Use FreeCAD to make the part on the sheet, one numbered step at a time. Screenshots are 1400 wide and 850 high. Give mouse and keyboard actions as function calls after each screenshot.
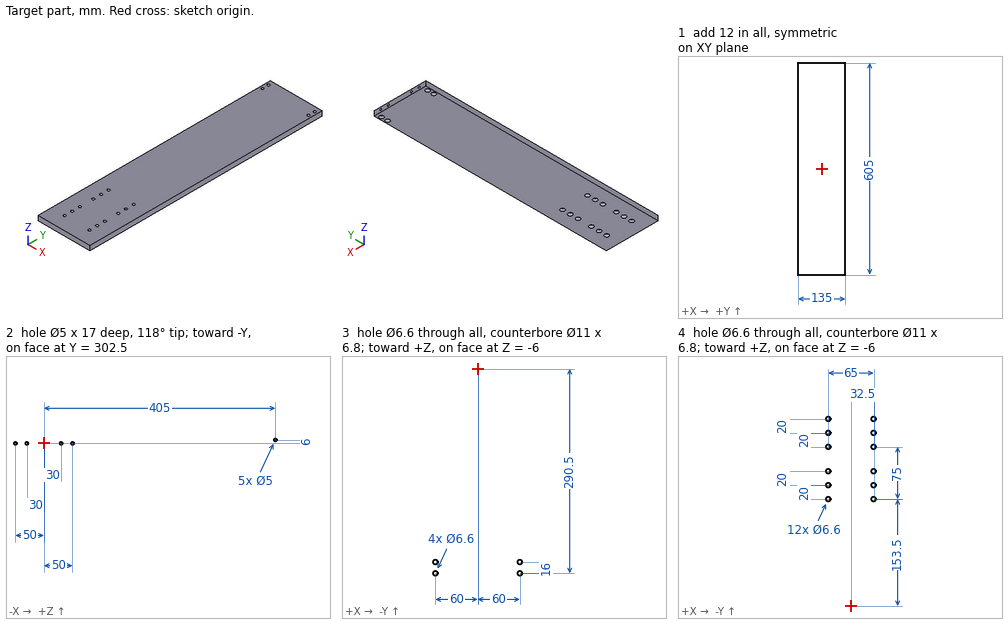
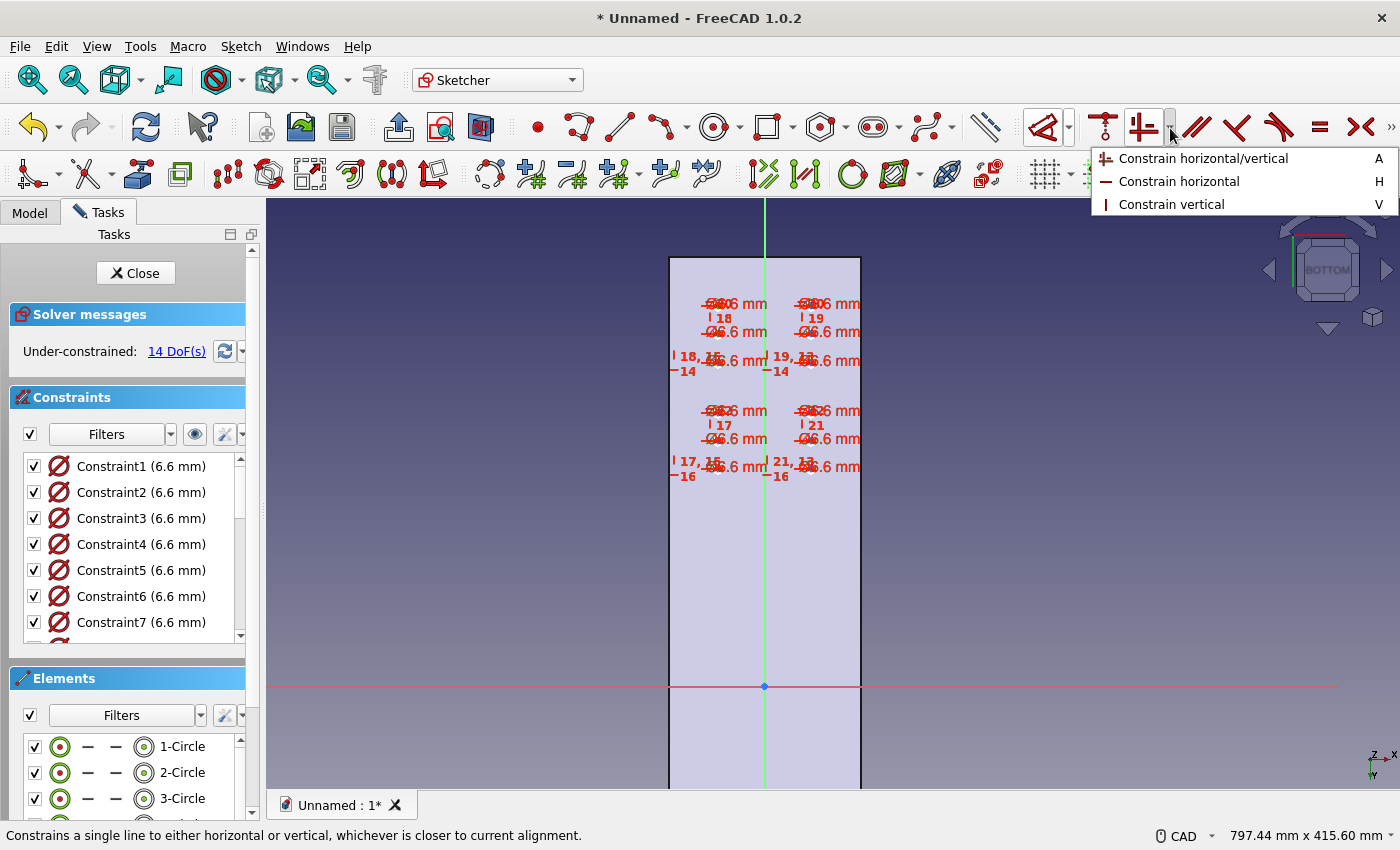
click(1245, 204)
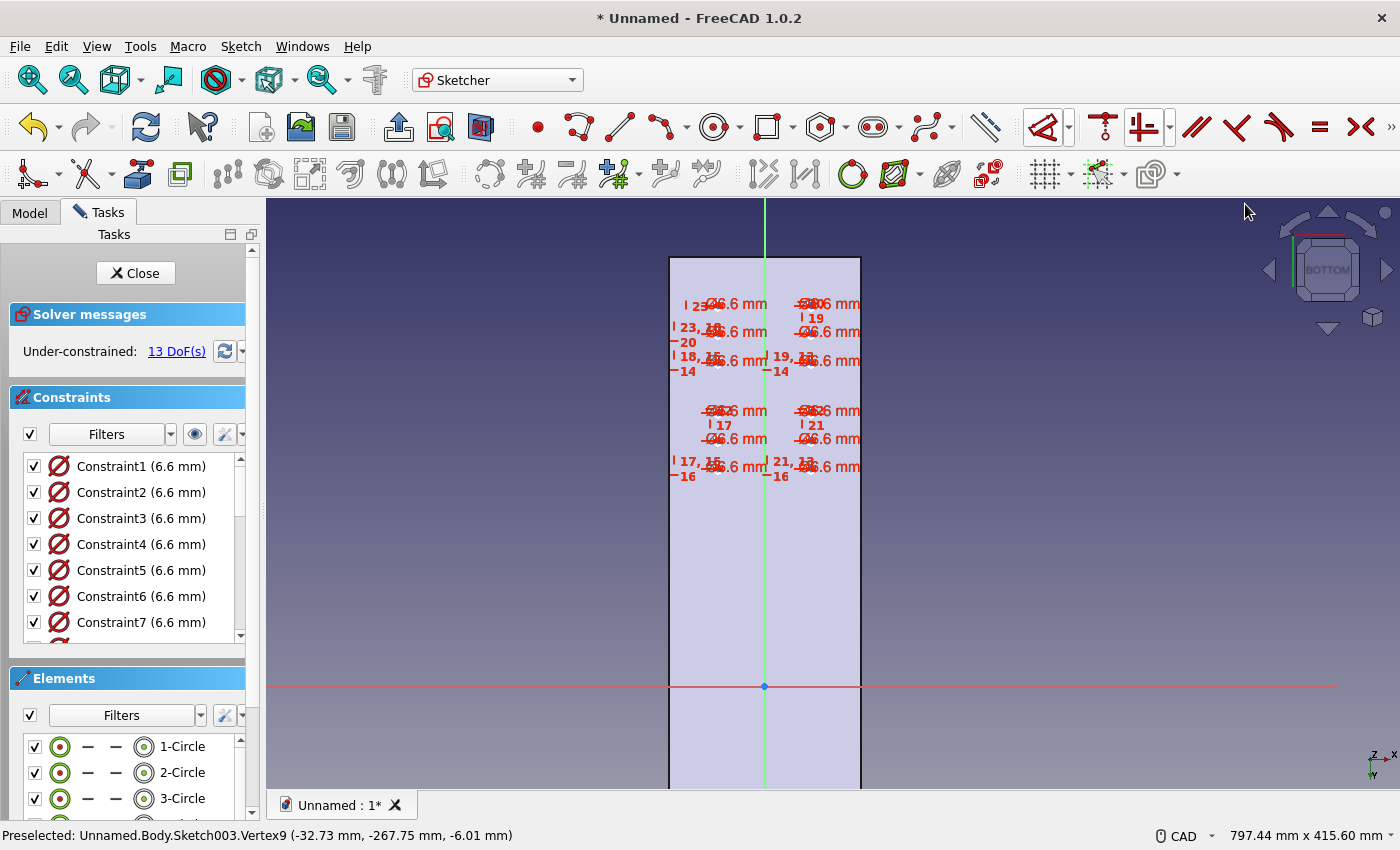
click(718, 441)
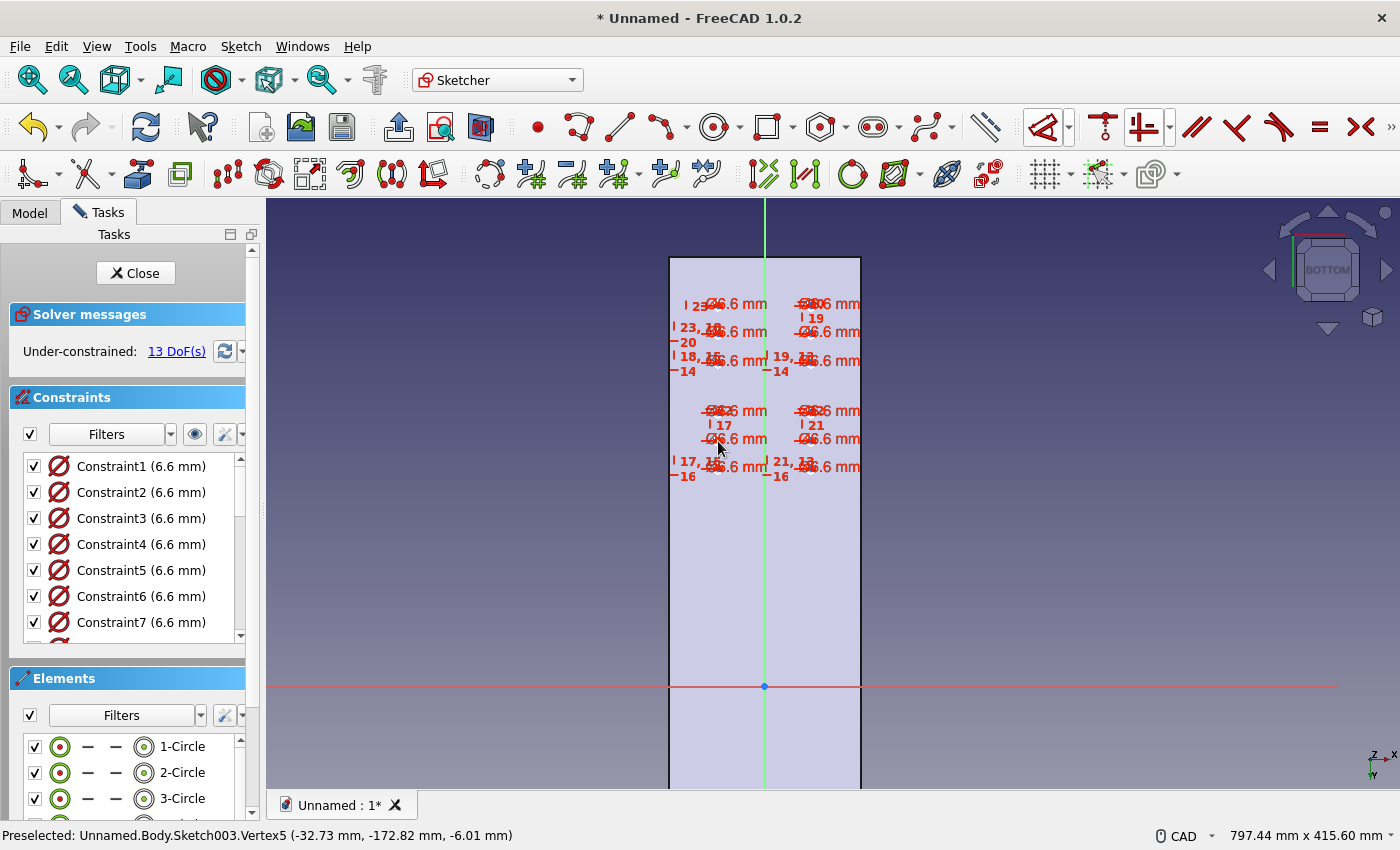
click(718, 413)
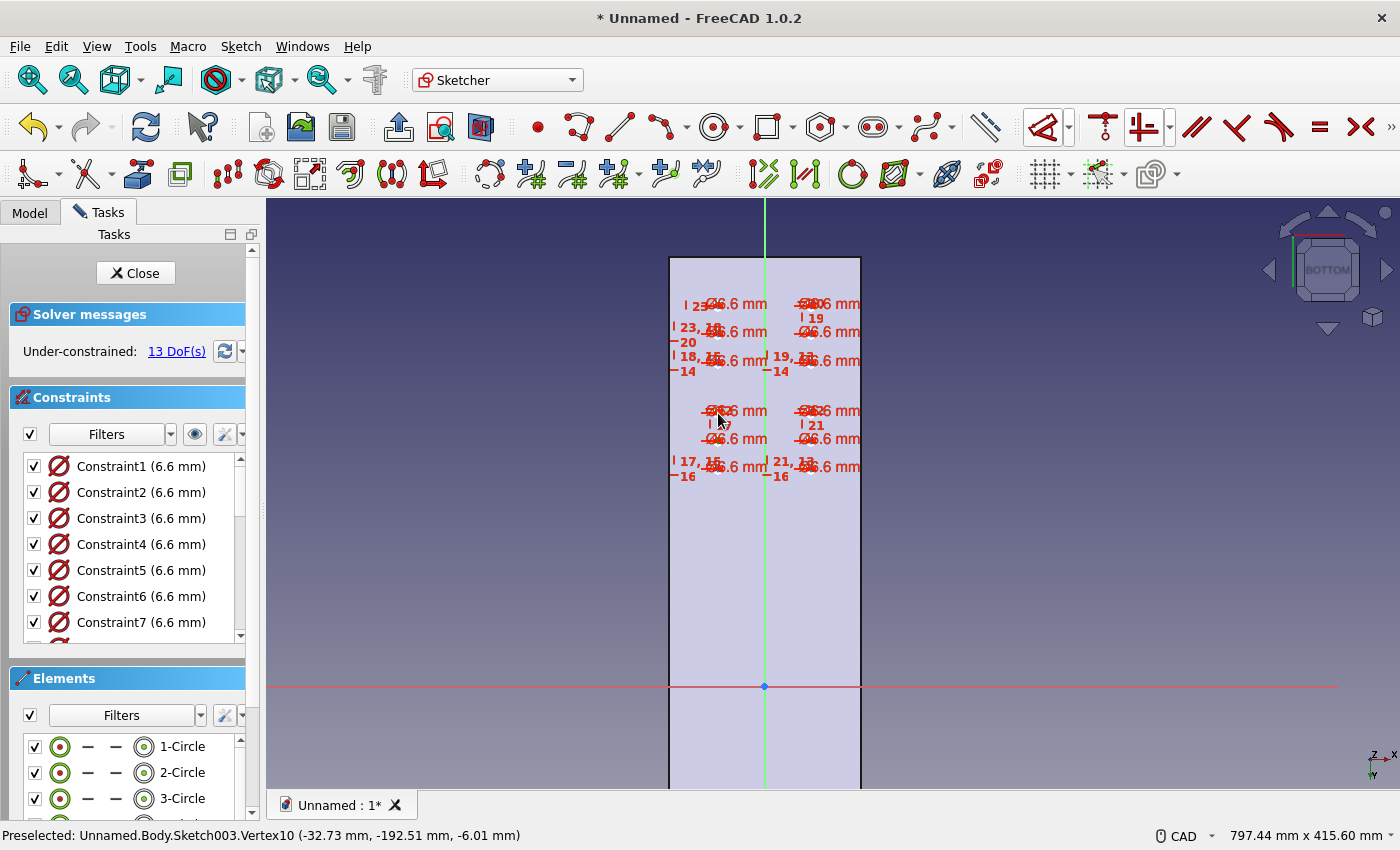
click(1170, 128)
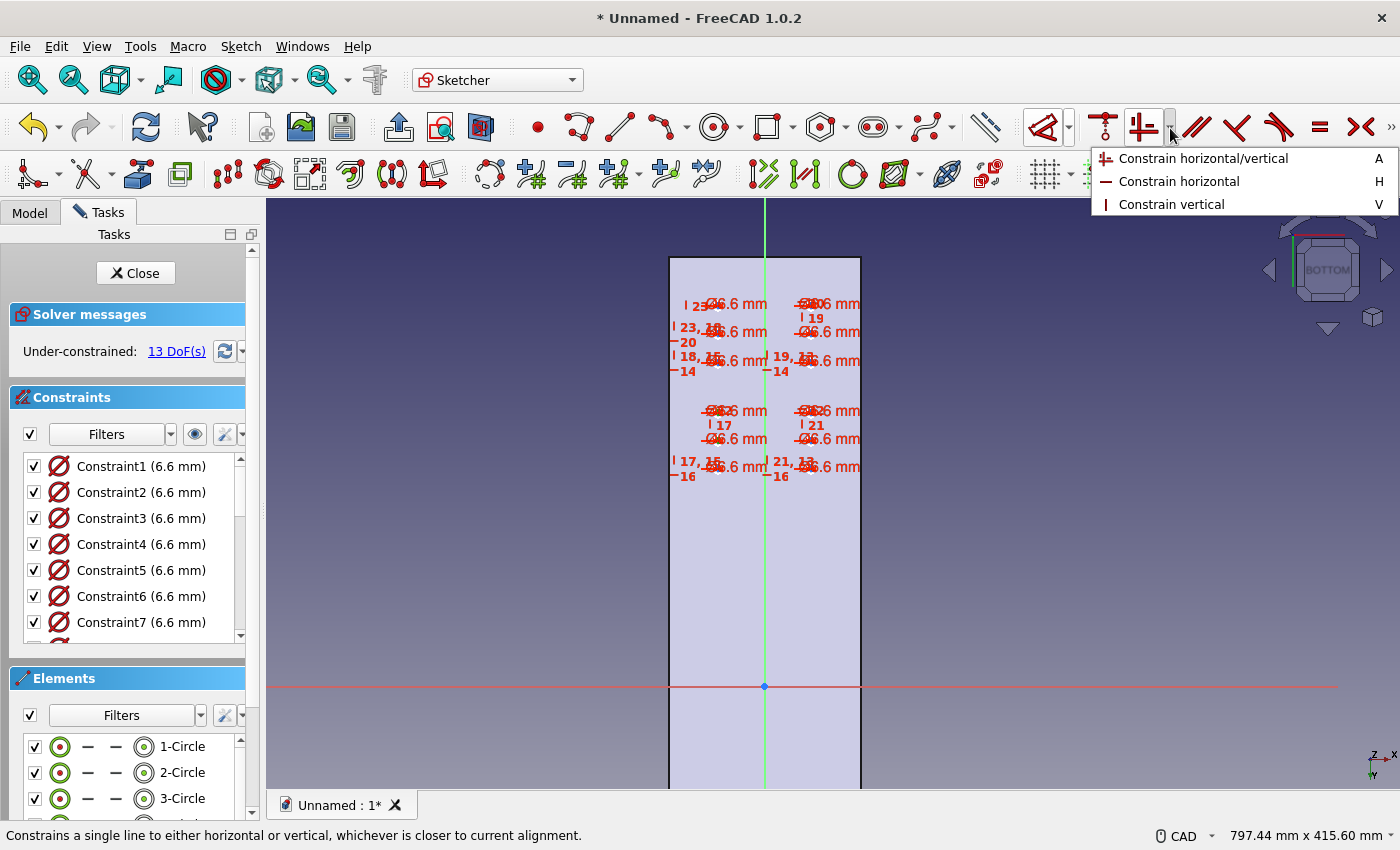
click(1245, 204)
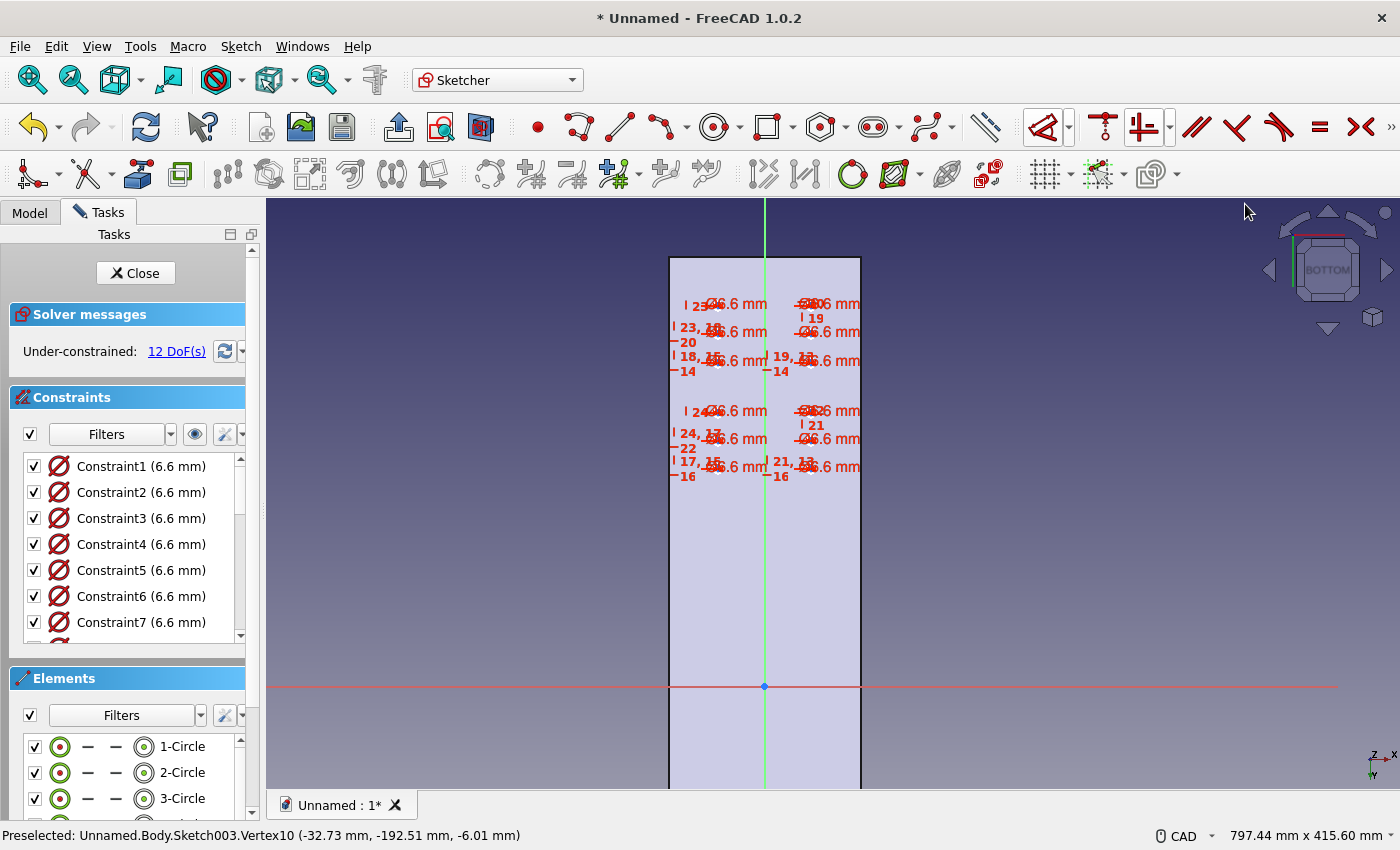
click(811, 441)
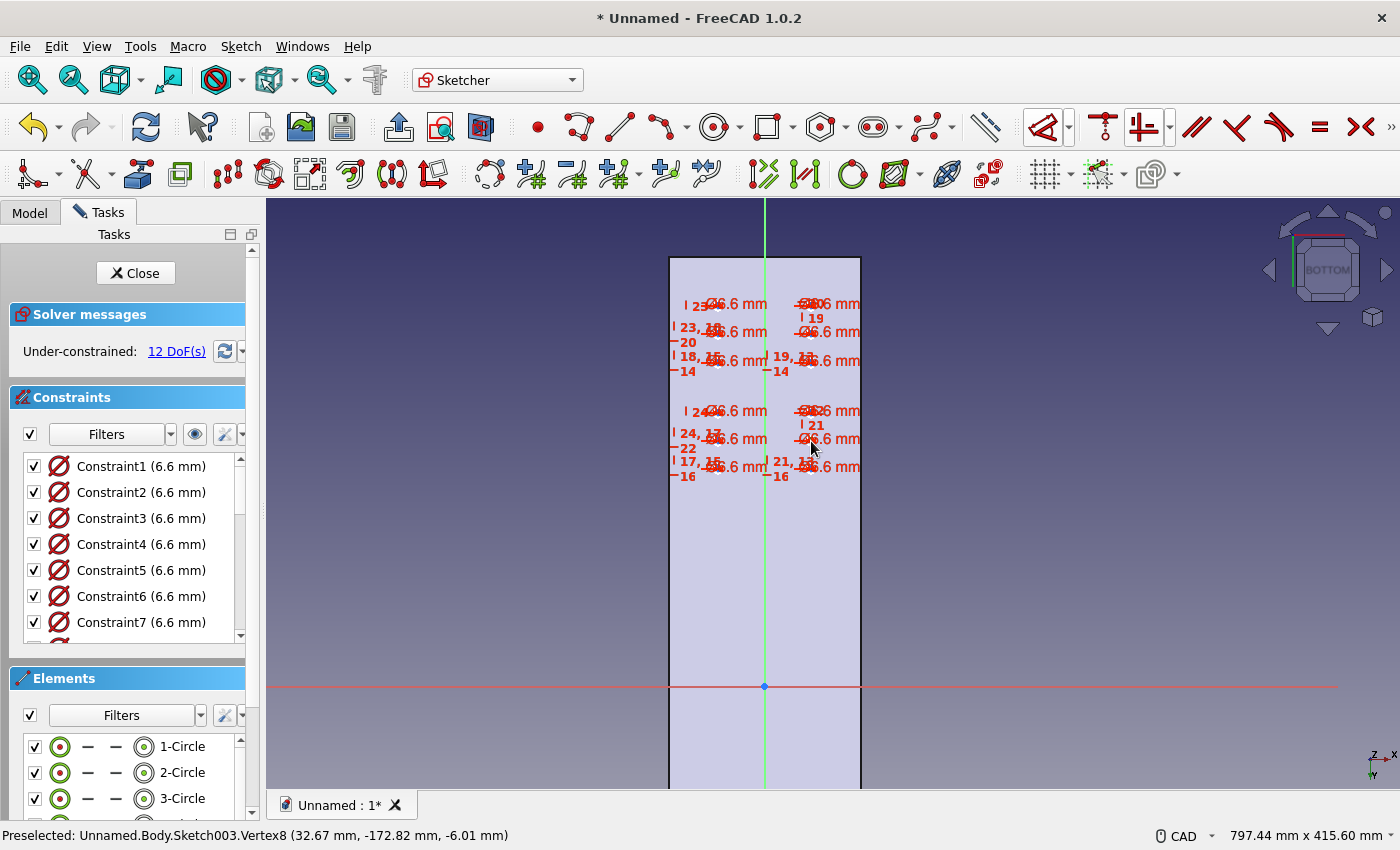
scroll(811, 413, up, 4)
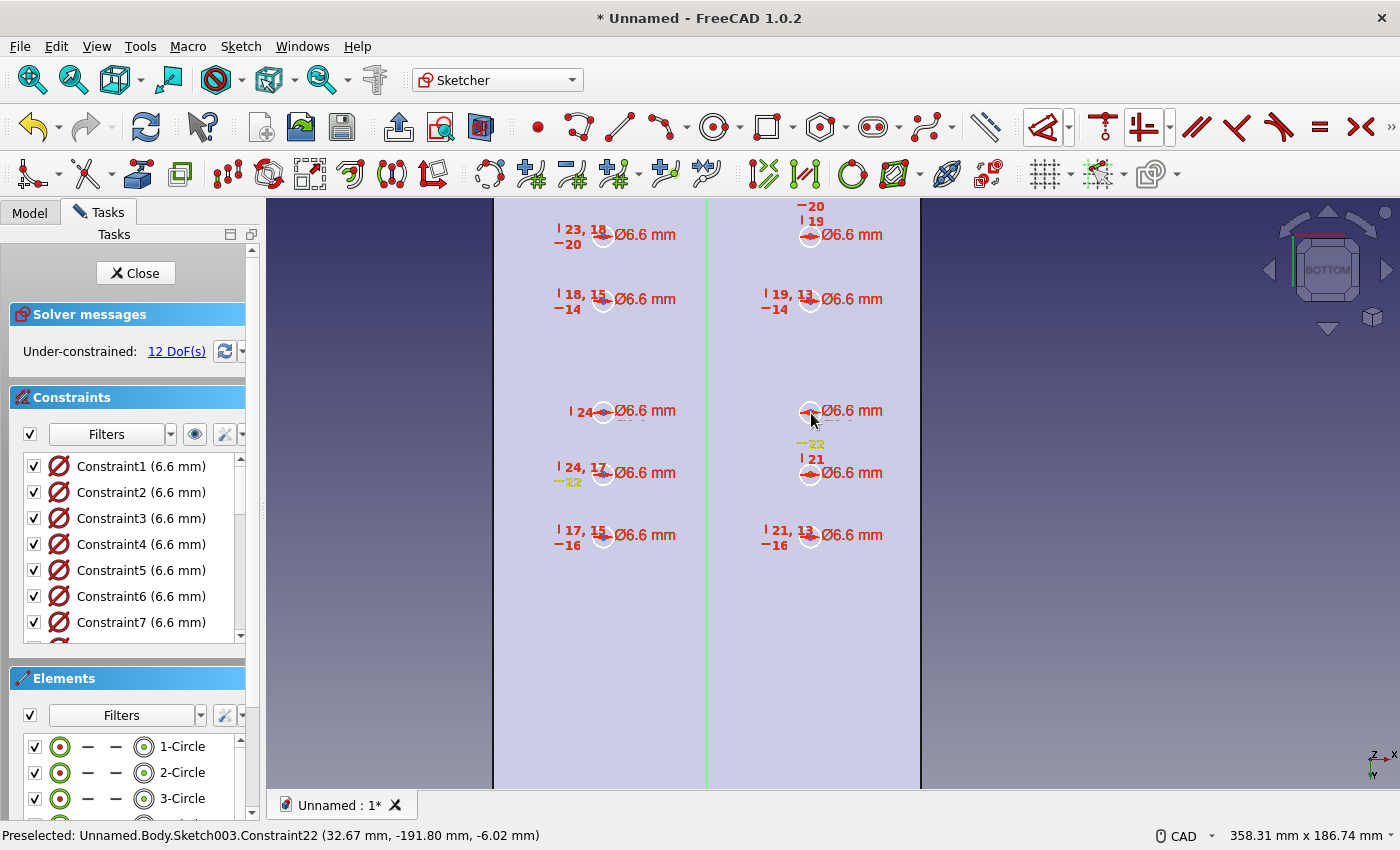
click(810, 413)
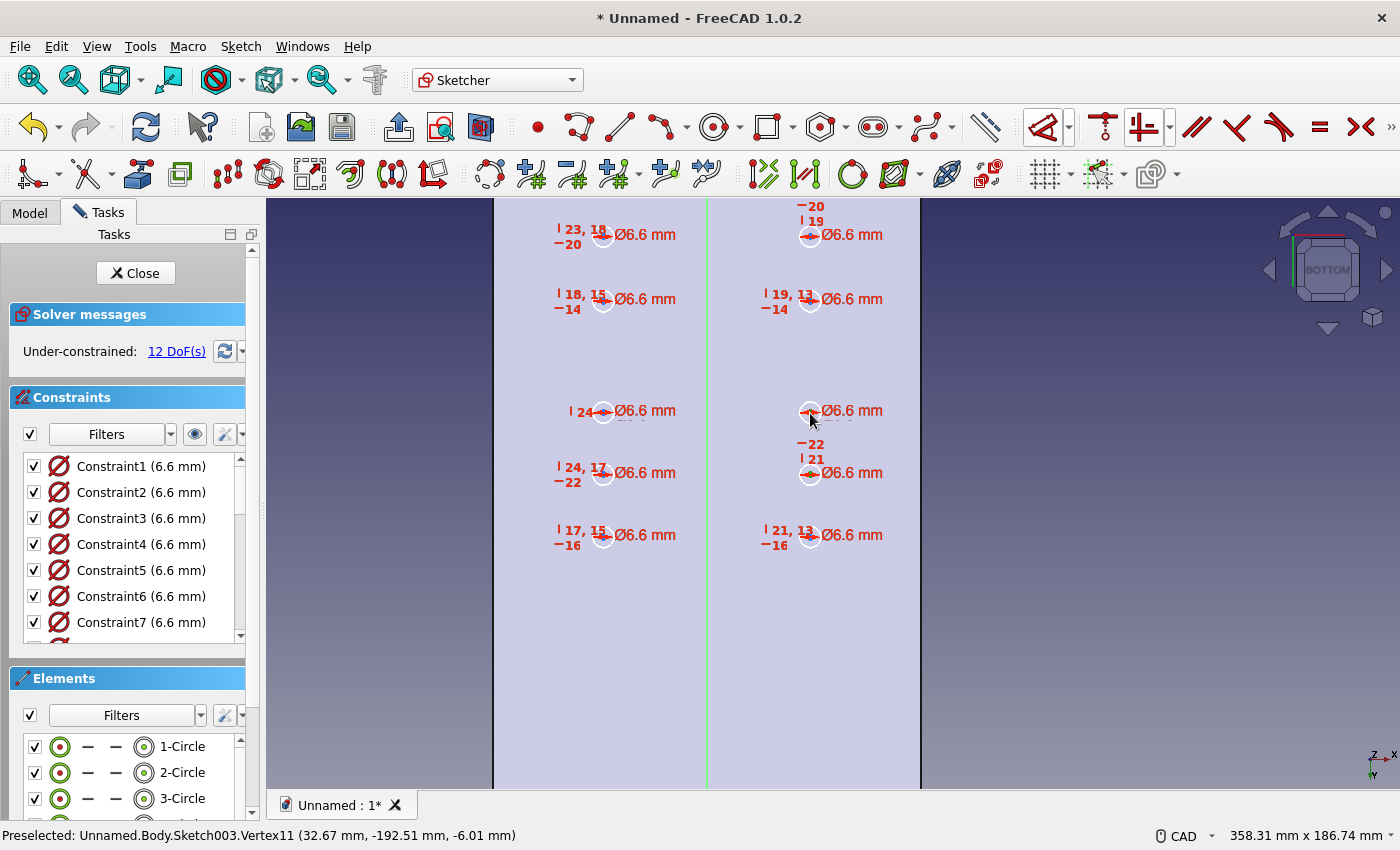
key(v)